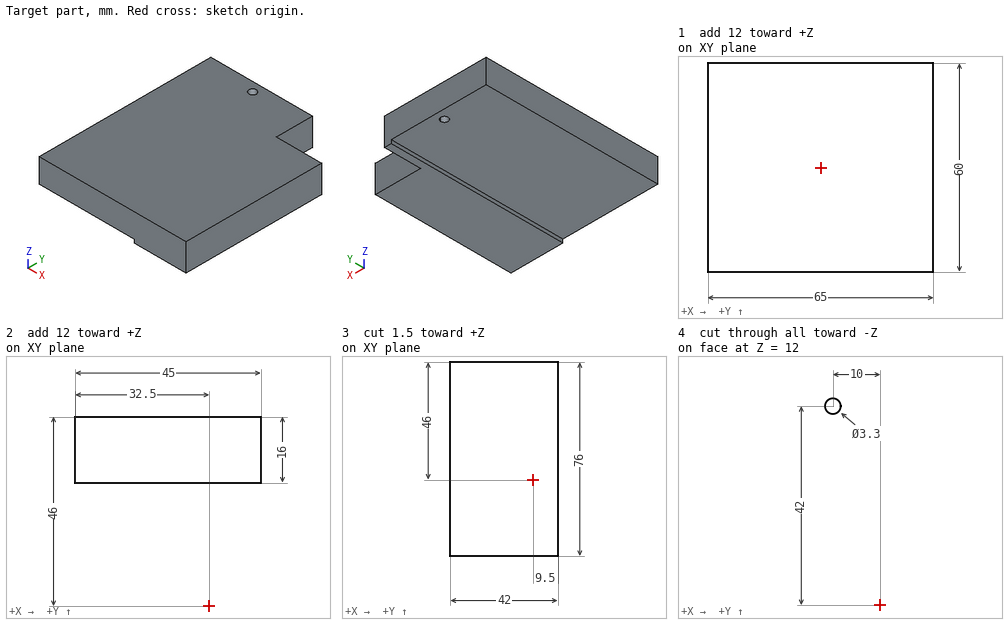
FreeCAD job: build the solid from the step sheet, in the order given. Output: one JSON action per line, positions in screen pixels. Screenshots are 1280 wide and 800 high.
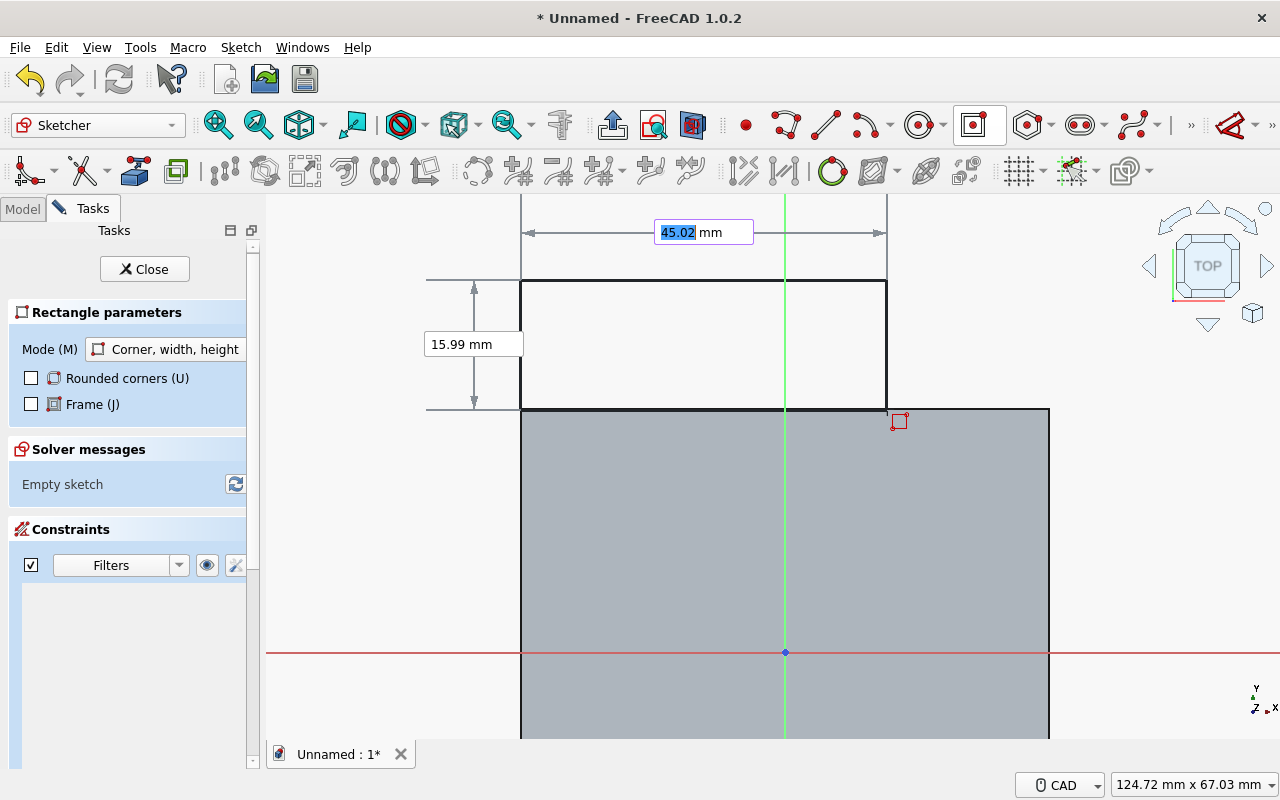
{"action": "type", "text": "45"}
{"action": "key", "text": "Tab"}
{"action": "type", "text": "16"}
{"action": "key", "text": "Return"}
{"action": "key", "text": "Escape"}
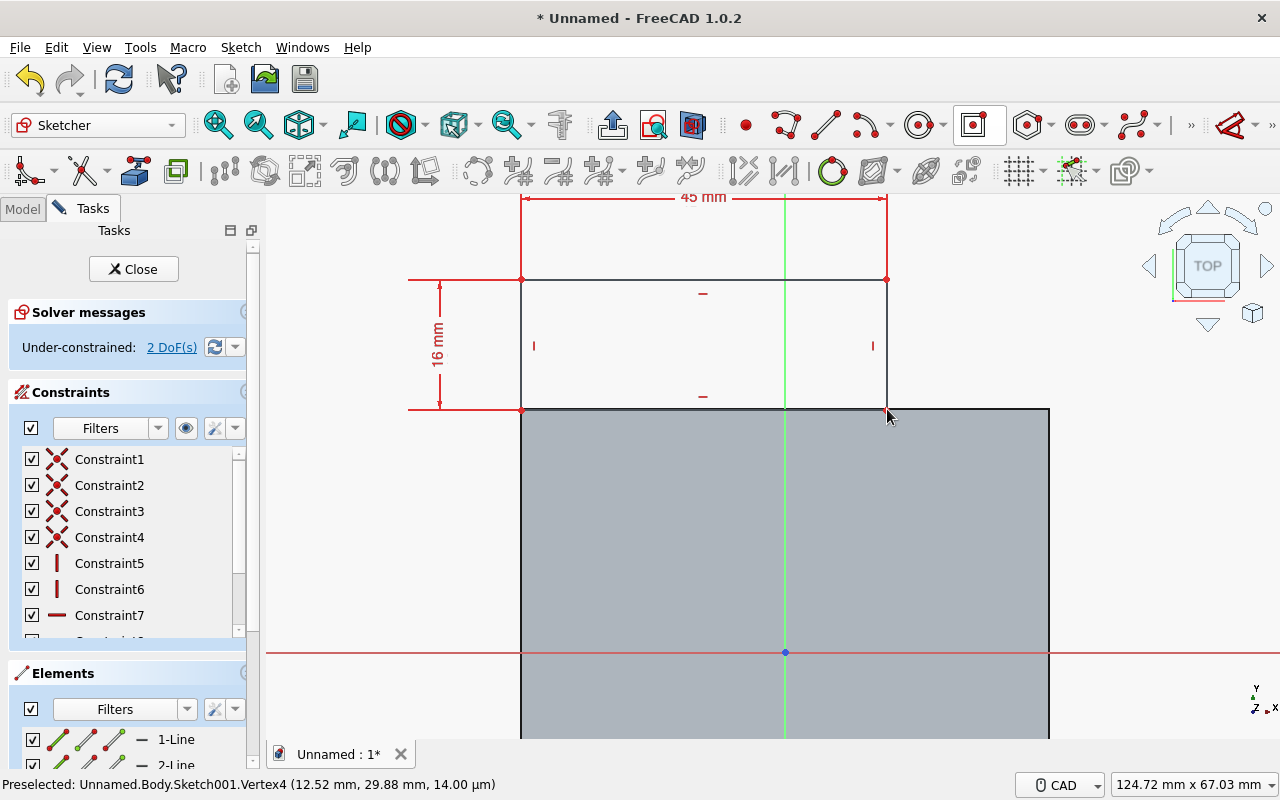
{"action": "left_click", "coordinate": [1230, 126]}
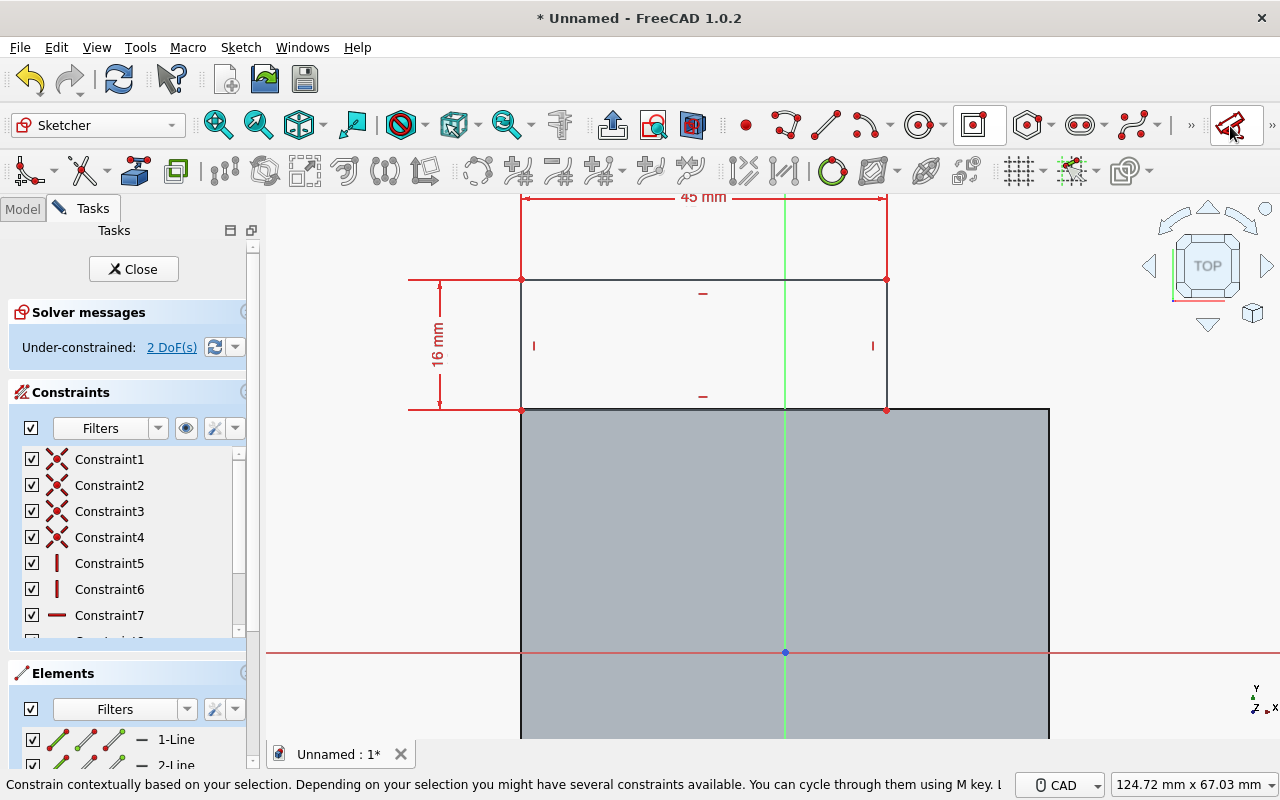
{"action": "left_click", "coordinate": [521, 280]}
{"action": "left_click", "coordinate": [487, 466]}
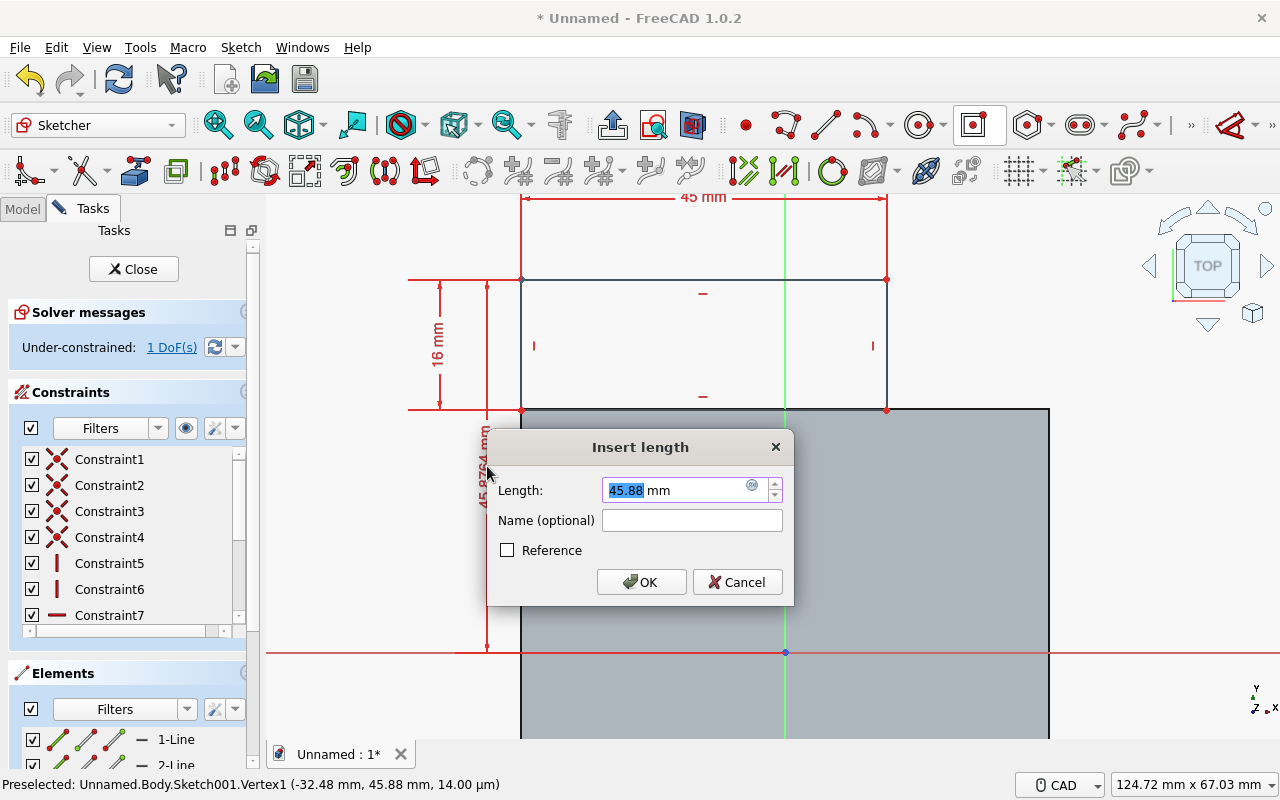
{"action": "type", "text": "46"}
{"action": "key", "text": "Return"}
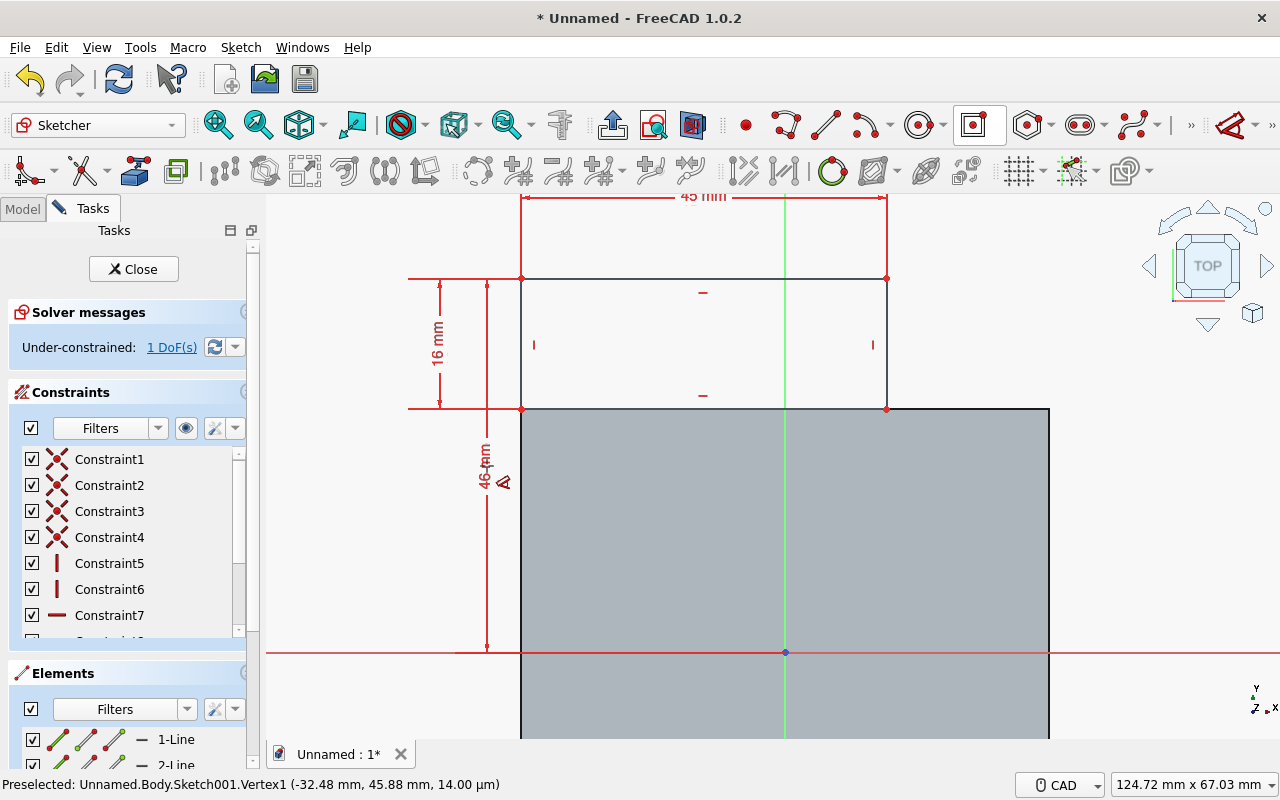
{"action": "left_click", "coordinate": [521, 279]}
{"action": "left_click", "coordinate": [653, 687]}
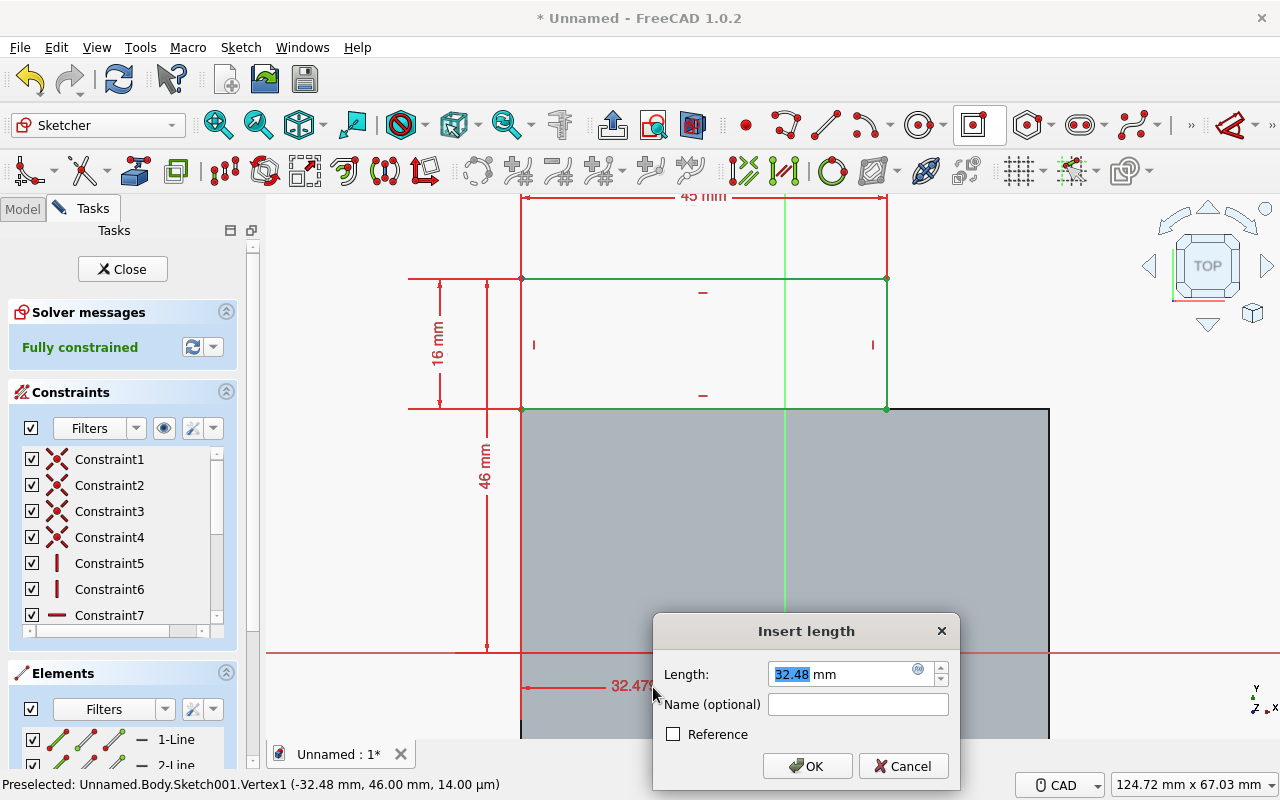
{"action": "type", "text": "32.5"}
{"action": "key", "text": "Return"}
{"action": "key", "text": "Escape"}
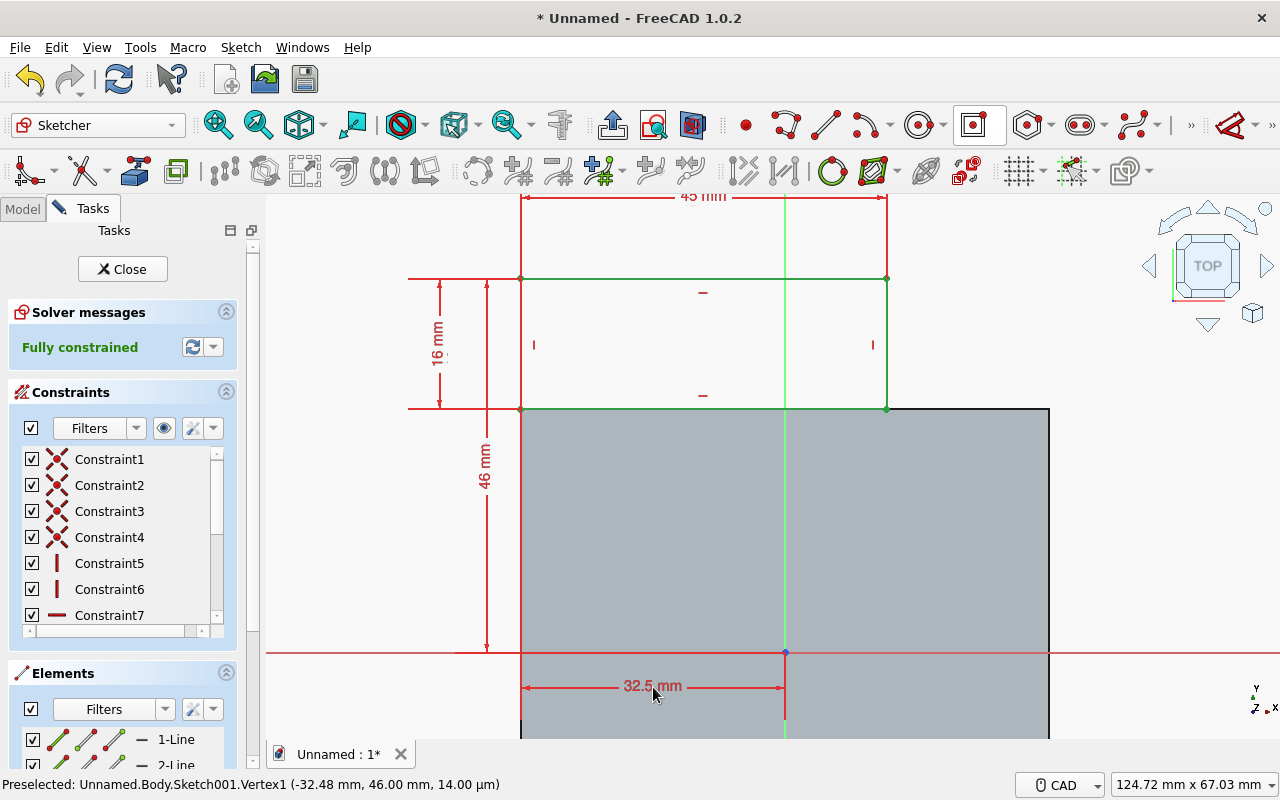
{"action": "left_click", "coordinate": [123, 269]}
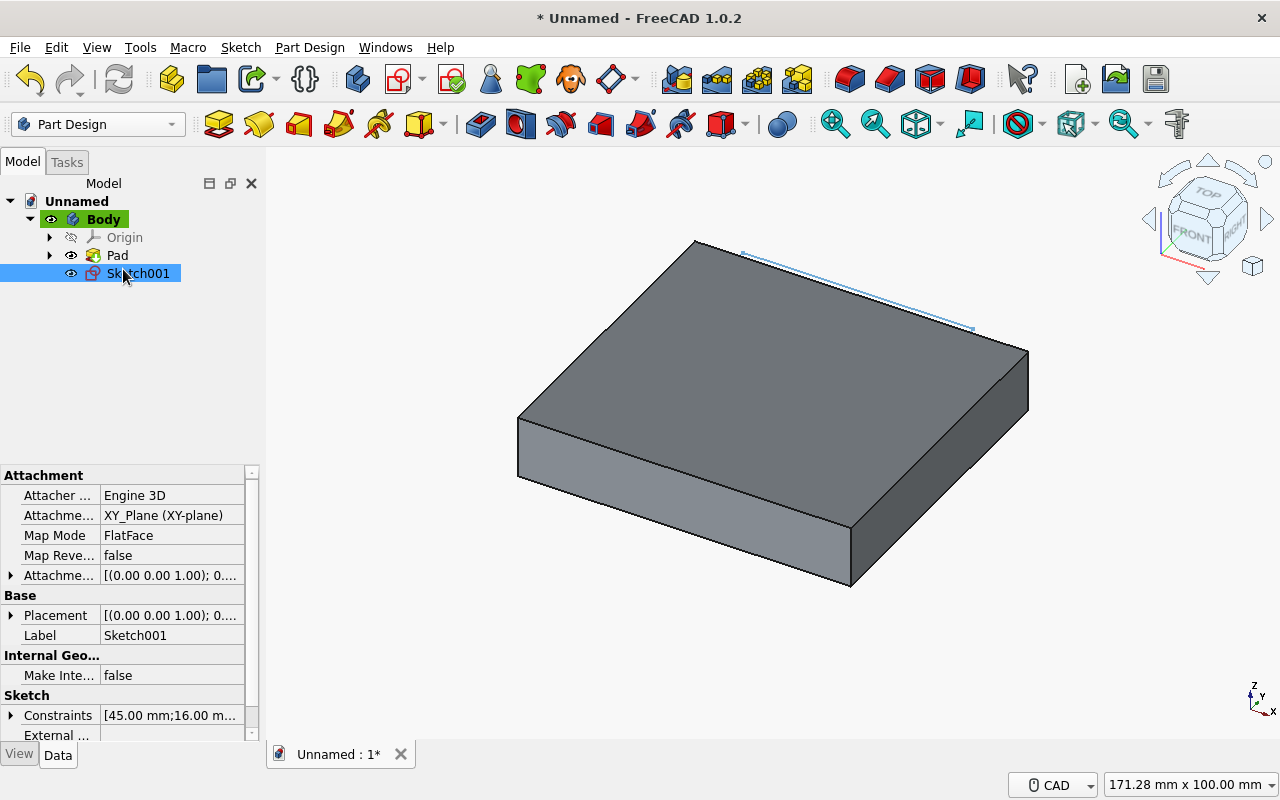
{"action": "left_click", "coordinate": [220, 124]}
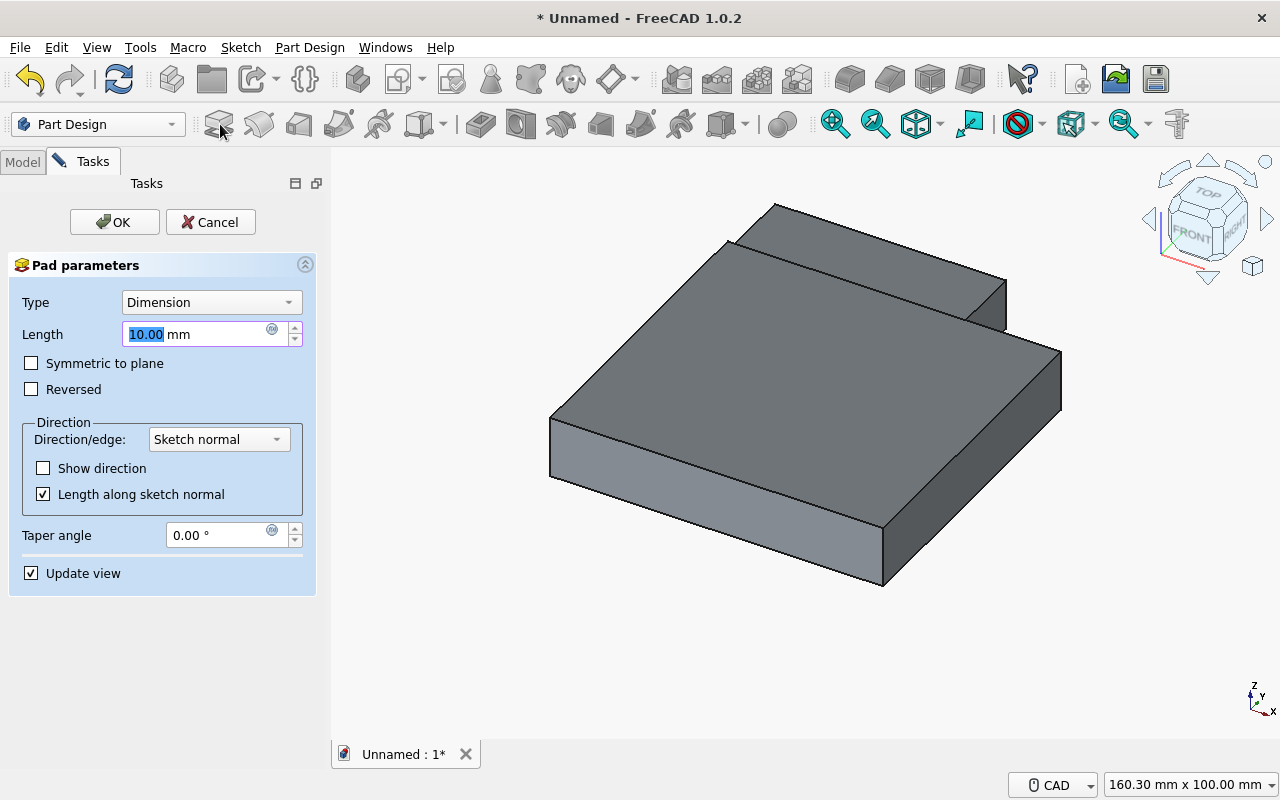
{"action": "type", "text": "12"}
{"action": "key", "text": "Tab"}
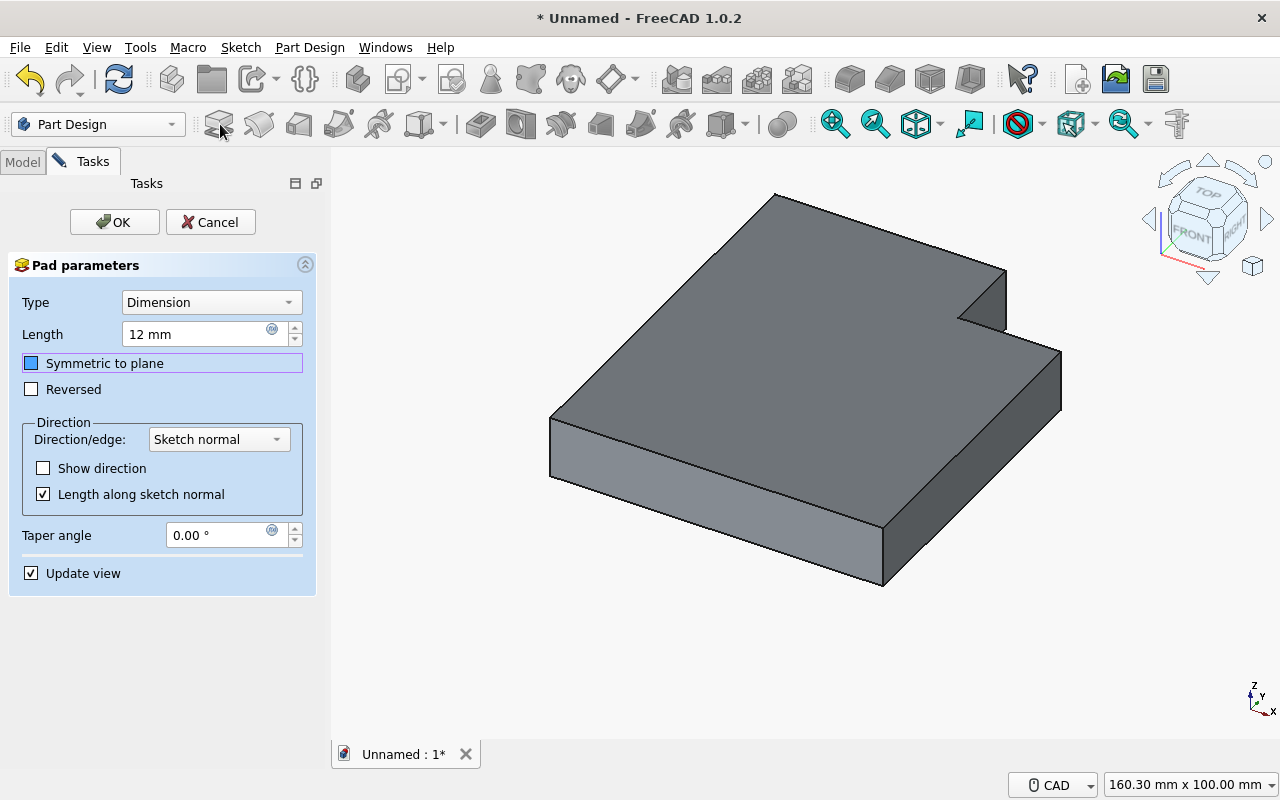
{"action": "left_click", "coordinate": [115, 222]}